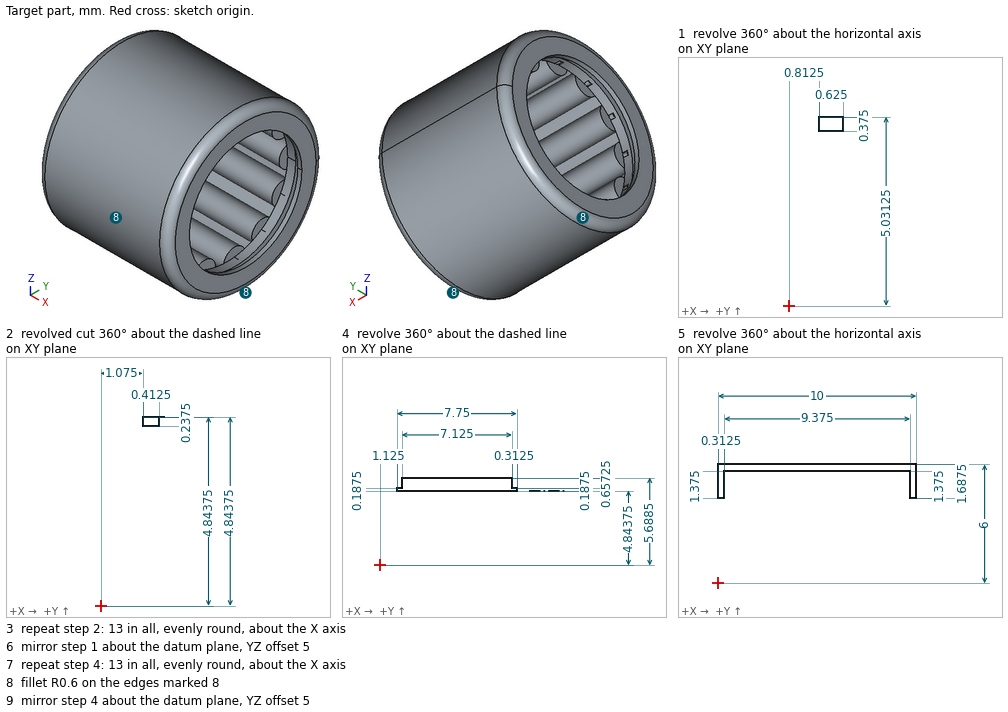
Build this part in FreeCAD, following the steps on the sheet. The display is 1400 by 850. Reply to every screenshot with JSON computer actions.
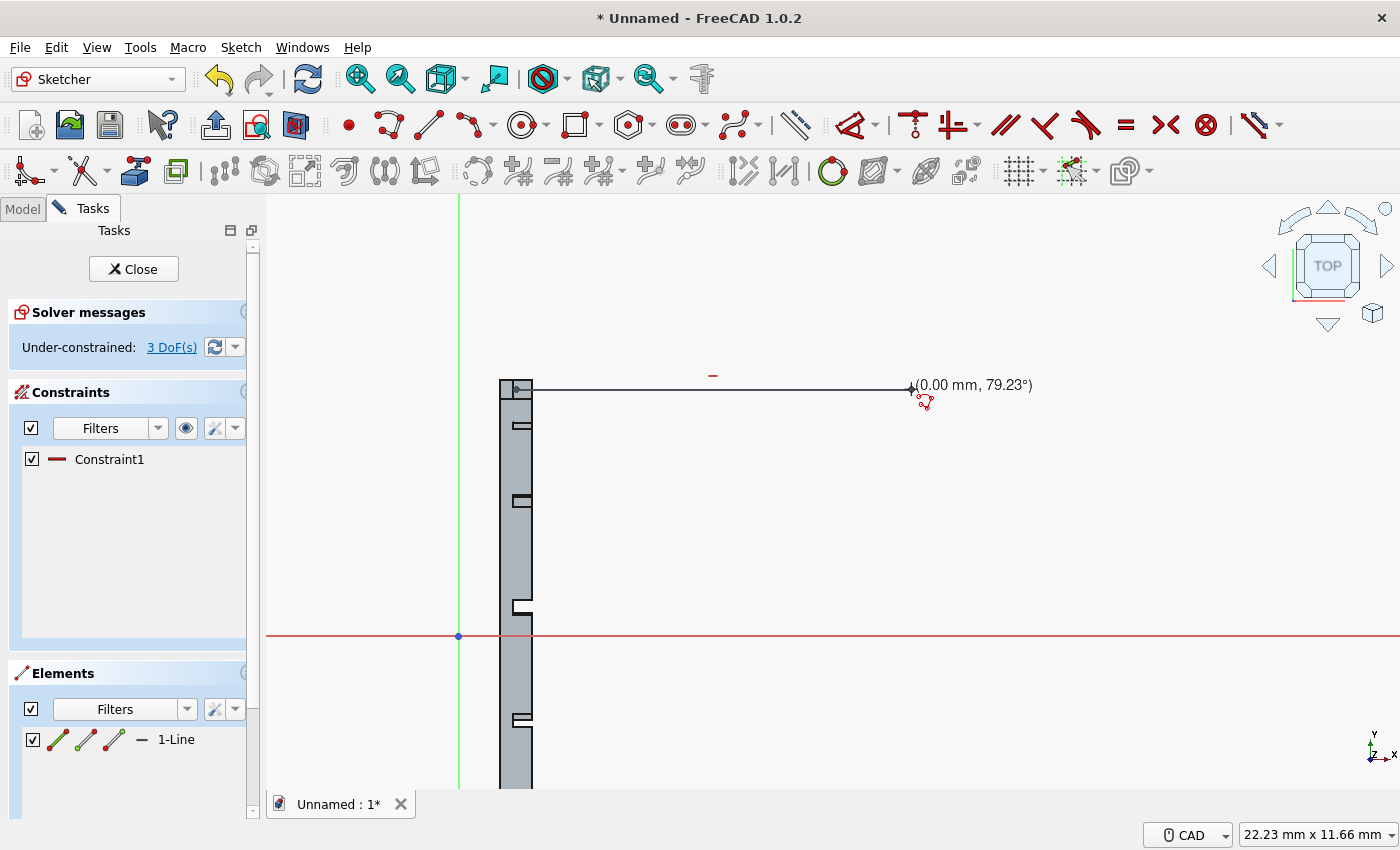
{"action": "scroll", "coordinate": [911, 380], "scroll_direction": "up", "scroll_amount": 3}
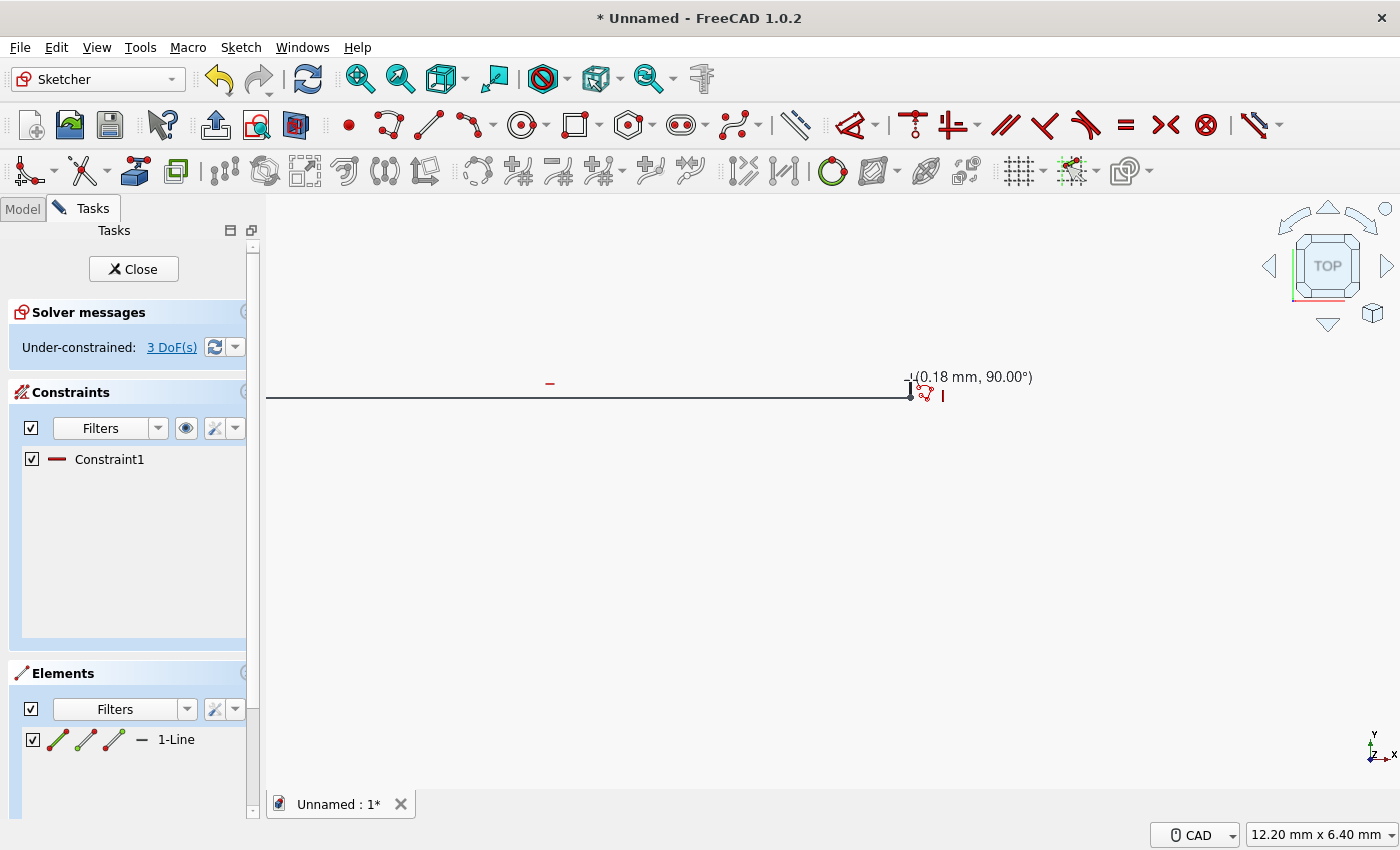
{"action": "left_click", "coordinate": [911, 379]}
{"action": "left_click", "coordinate": [882, 379]}
{"action": "left_click", "coordinate": [882, 318]}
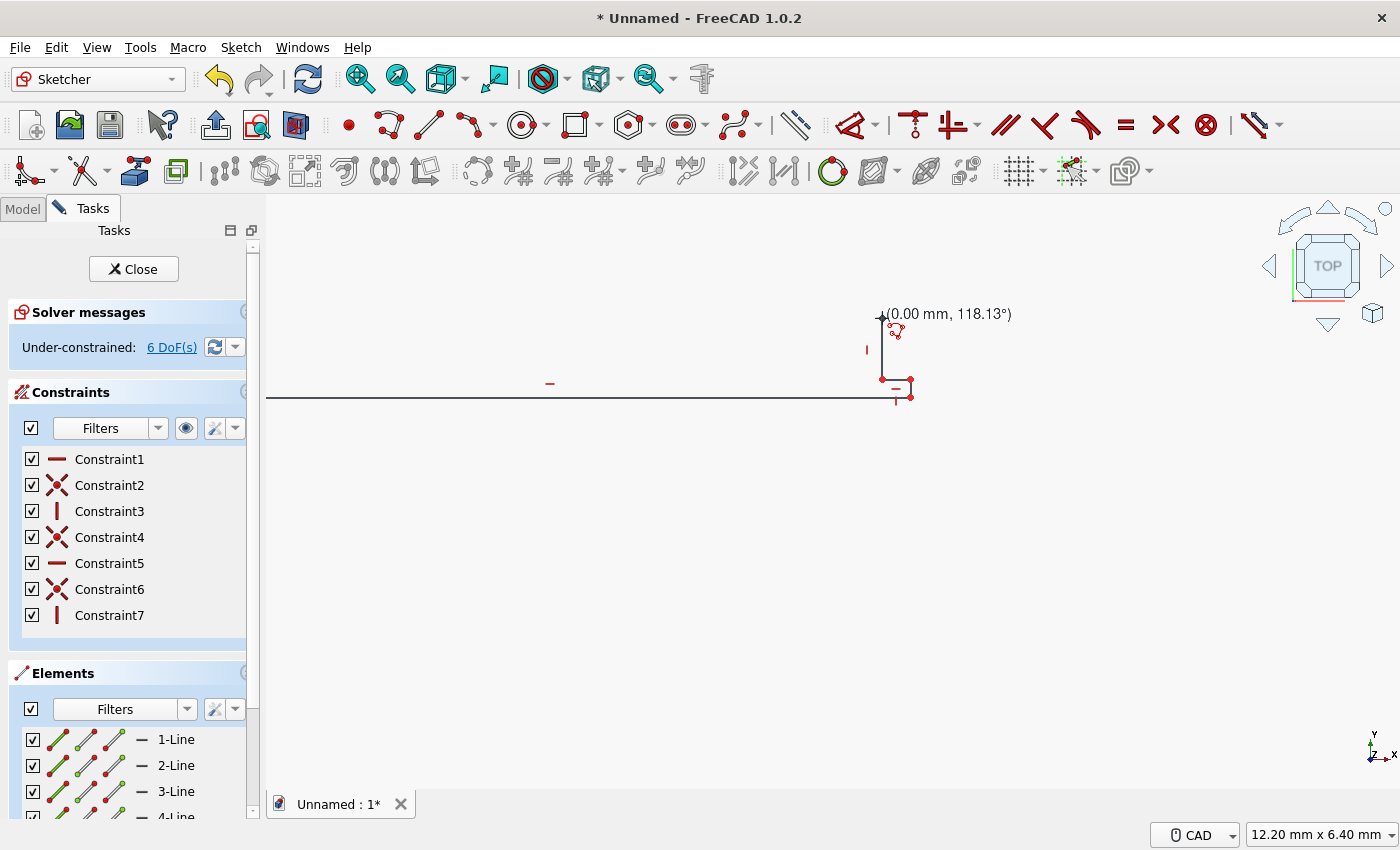
{"action": "scroll", "coordinate": [912, 381], "scroll_direction": "down", "scroll_amount": 3}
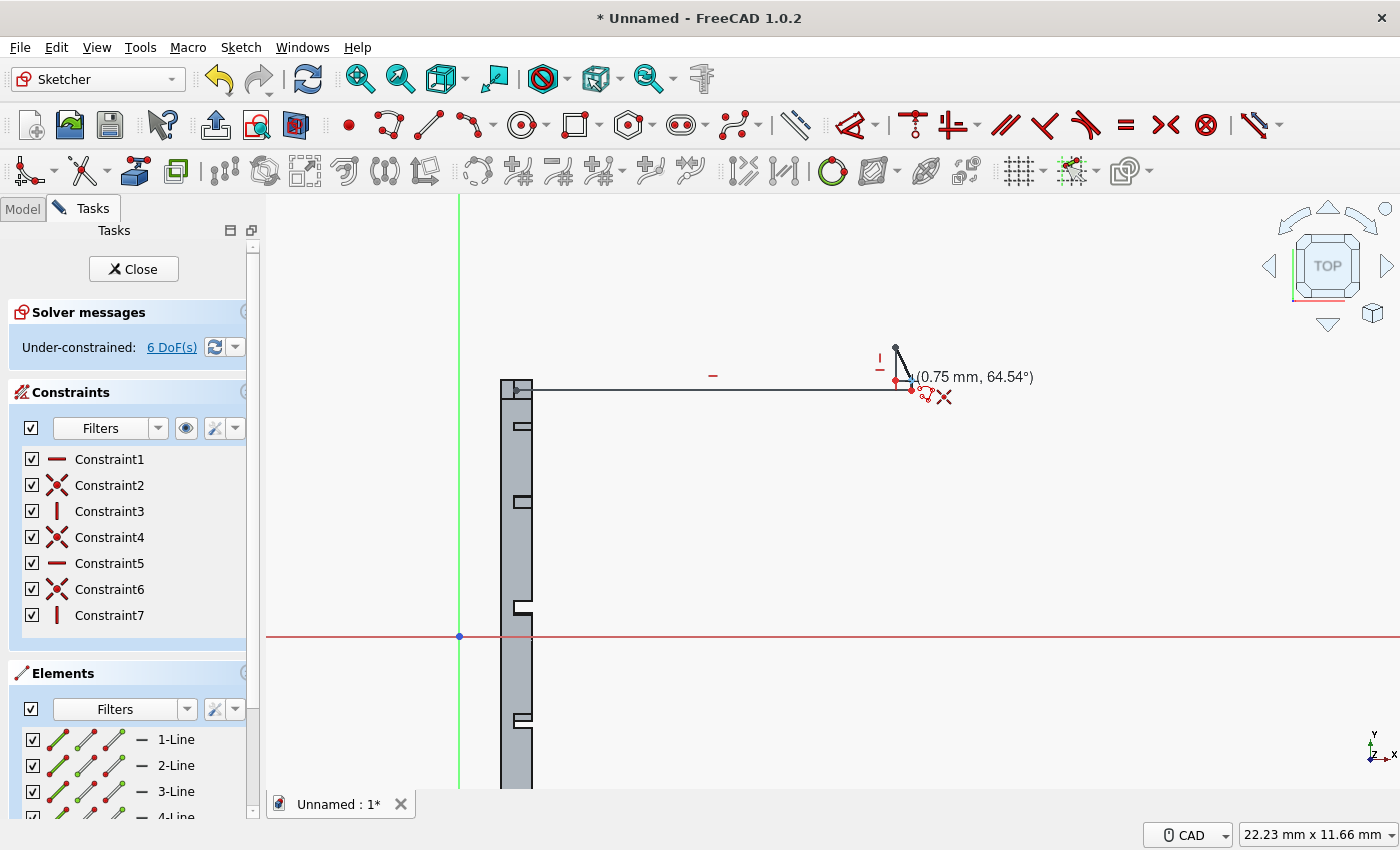
{"action": "left_click", "coordinate": [532, 347]}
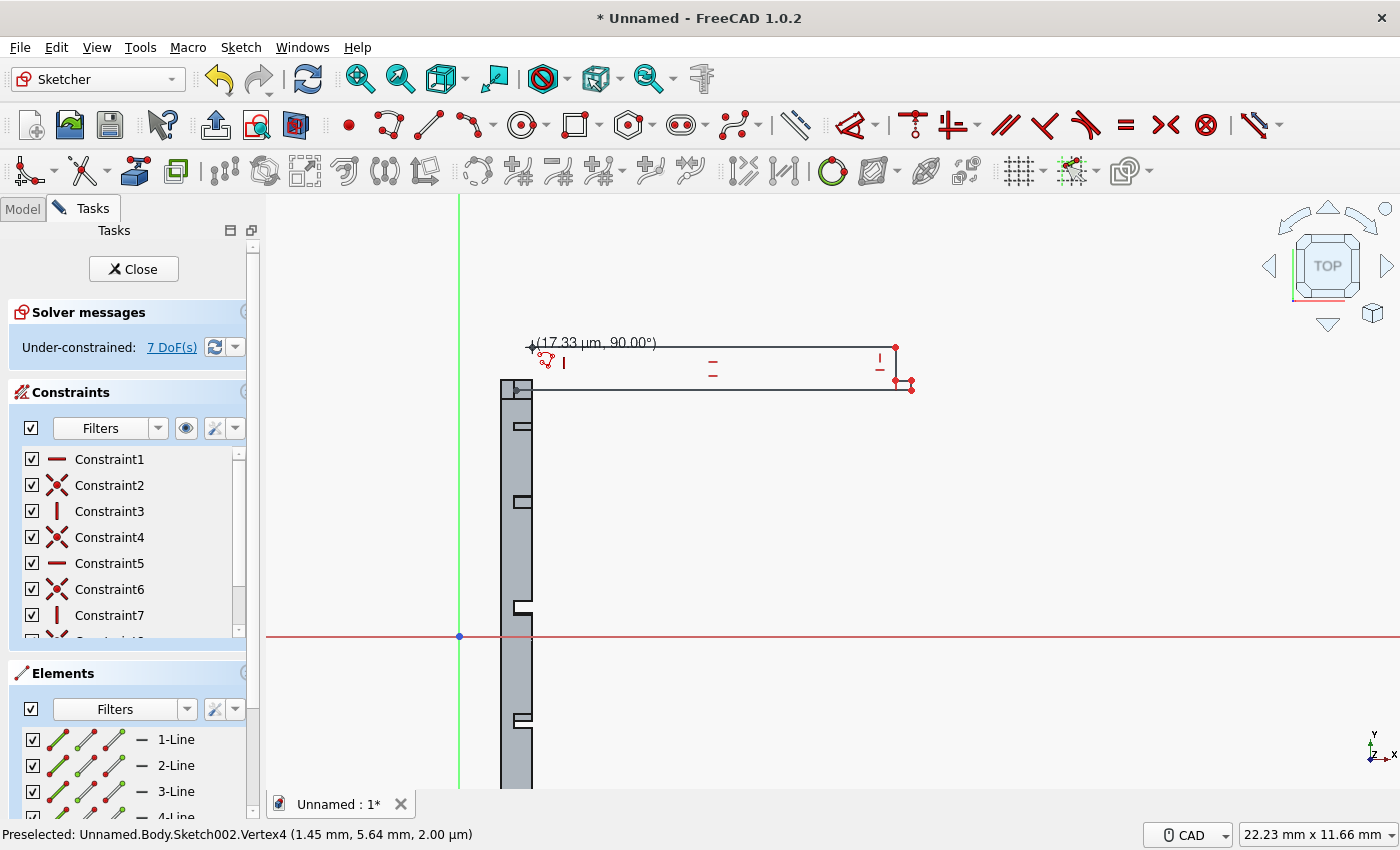
{"action": "scroll", "coordinate": [532, 380], "scroll_direction": "up", "scroll_amount": 3}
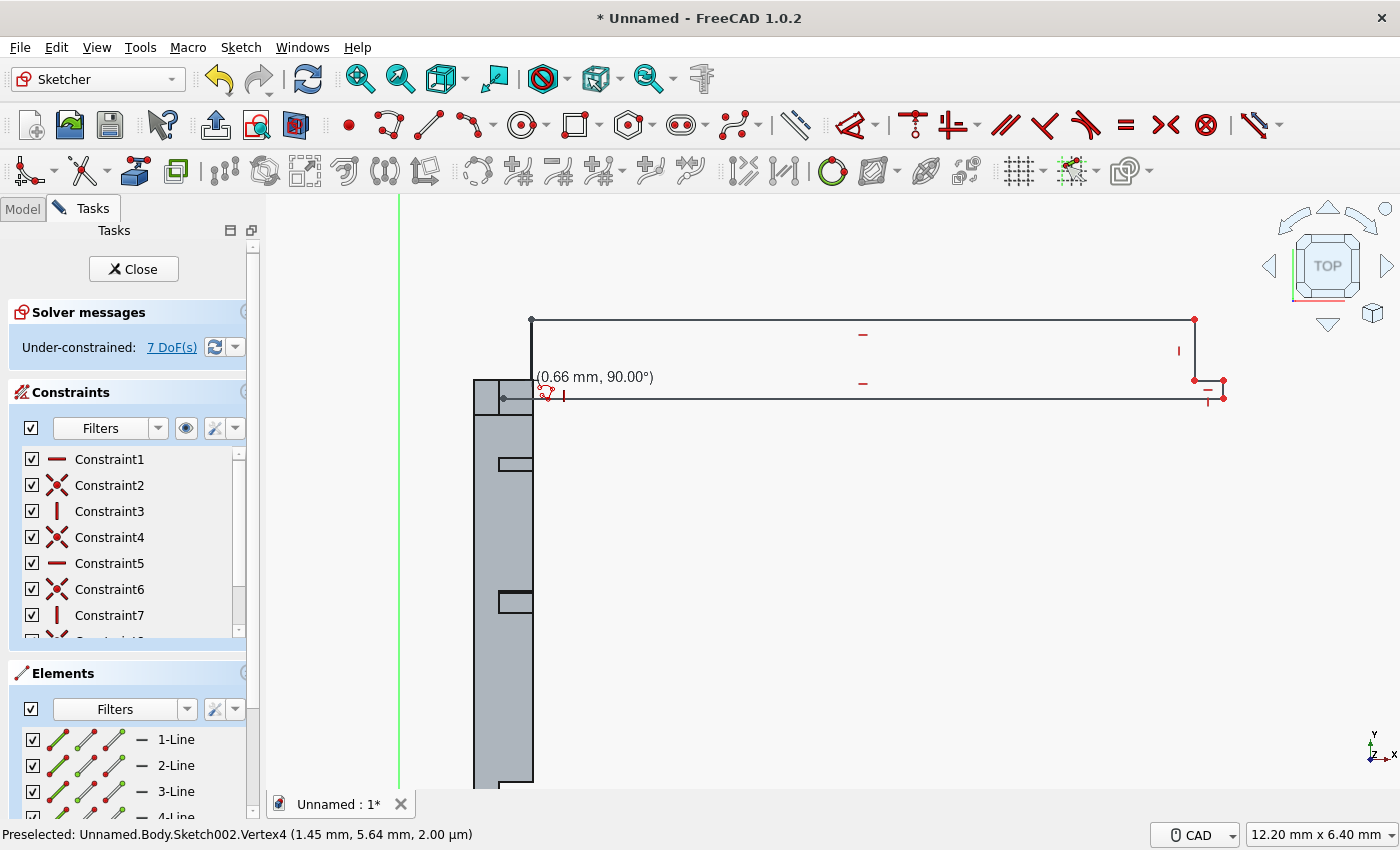
{"action": "left_click", "coordinate": [532, 380]}
{"action": "left_click", "coordinate": [503, 380]}
{"action": "left_click", "coordinate": [503, 399]}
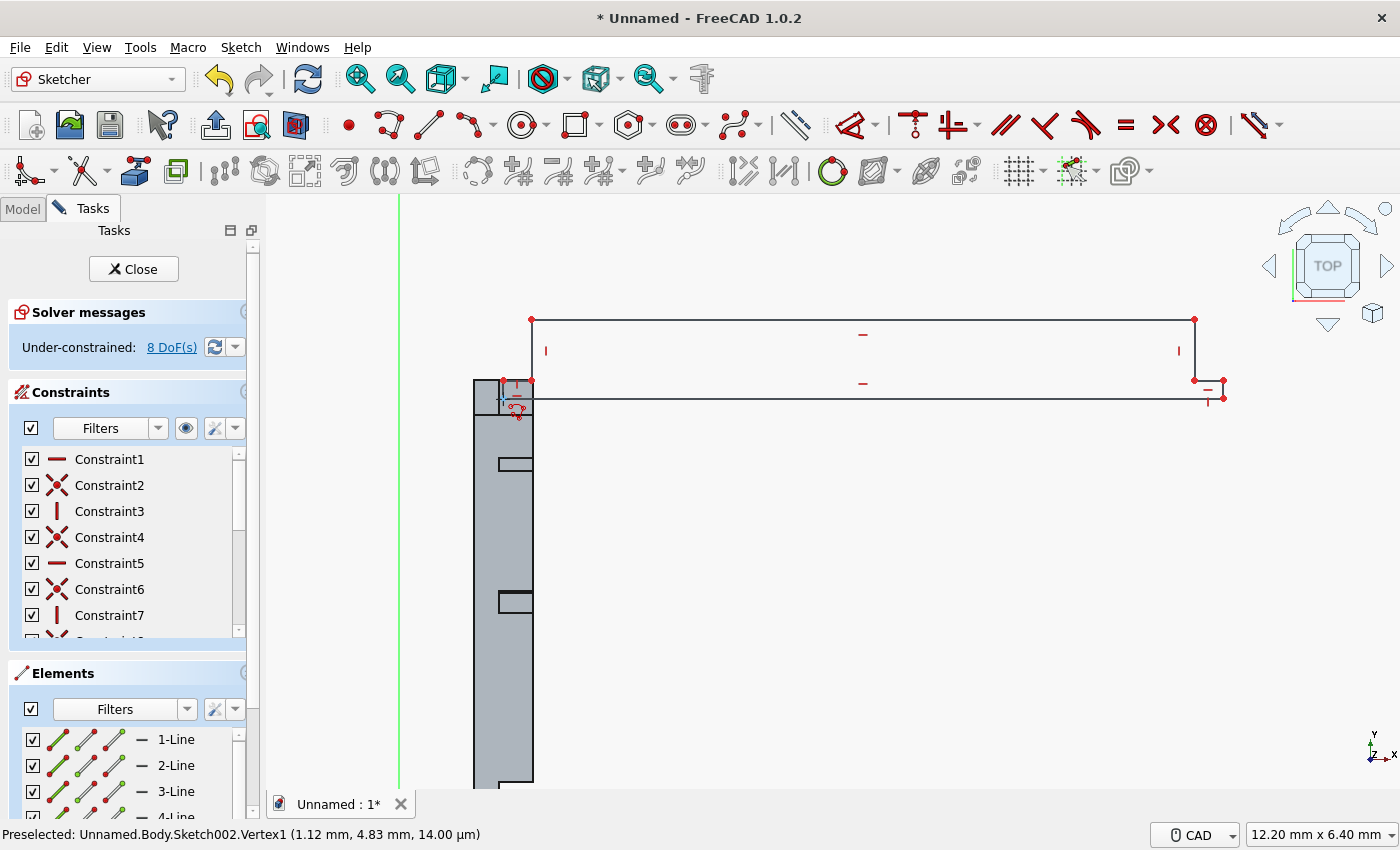
{"action": "left_click", "coordinate": [430, 126]}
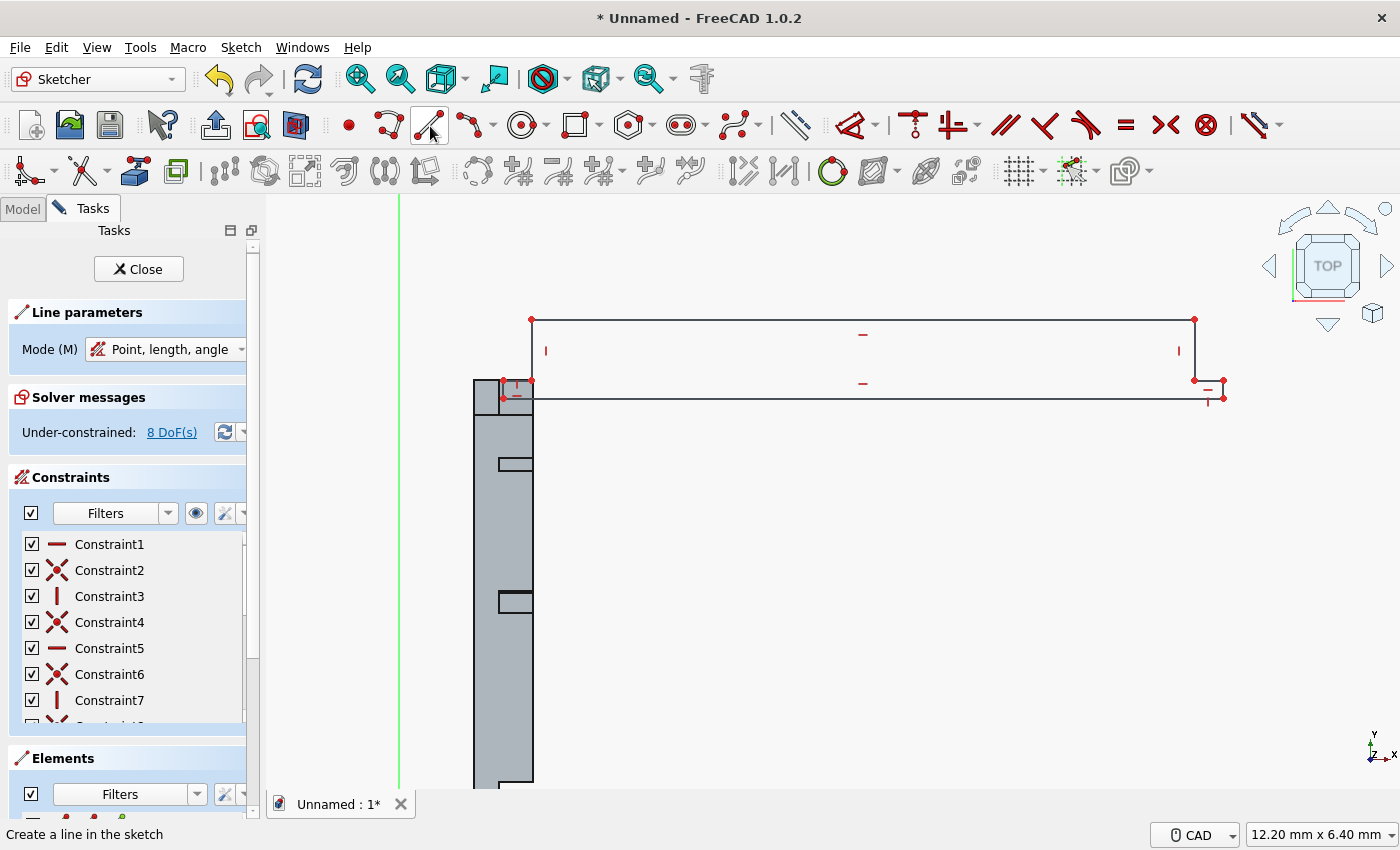
{"action": "scroll", "coordinate": [532, 380], "scroll_direction": "down", "scroll_amount": 3}